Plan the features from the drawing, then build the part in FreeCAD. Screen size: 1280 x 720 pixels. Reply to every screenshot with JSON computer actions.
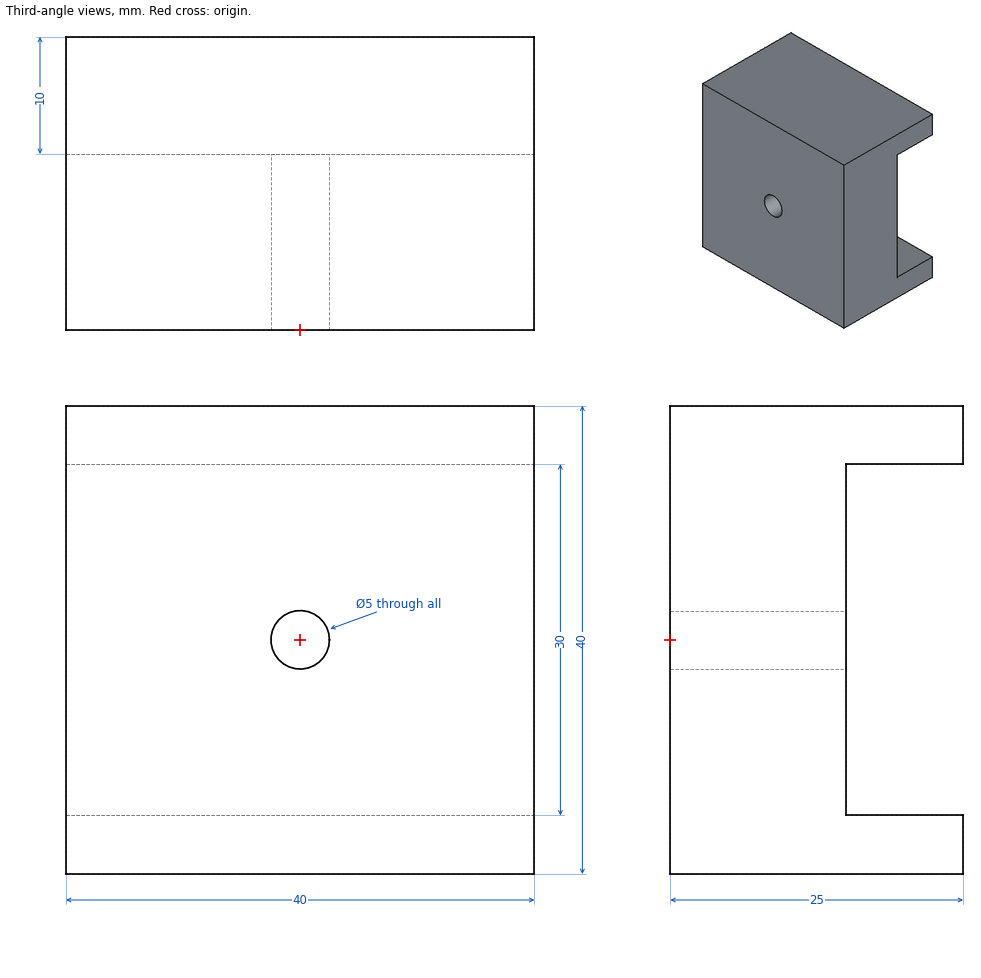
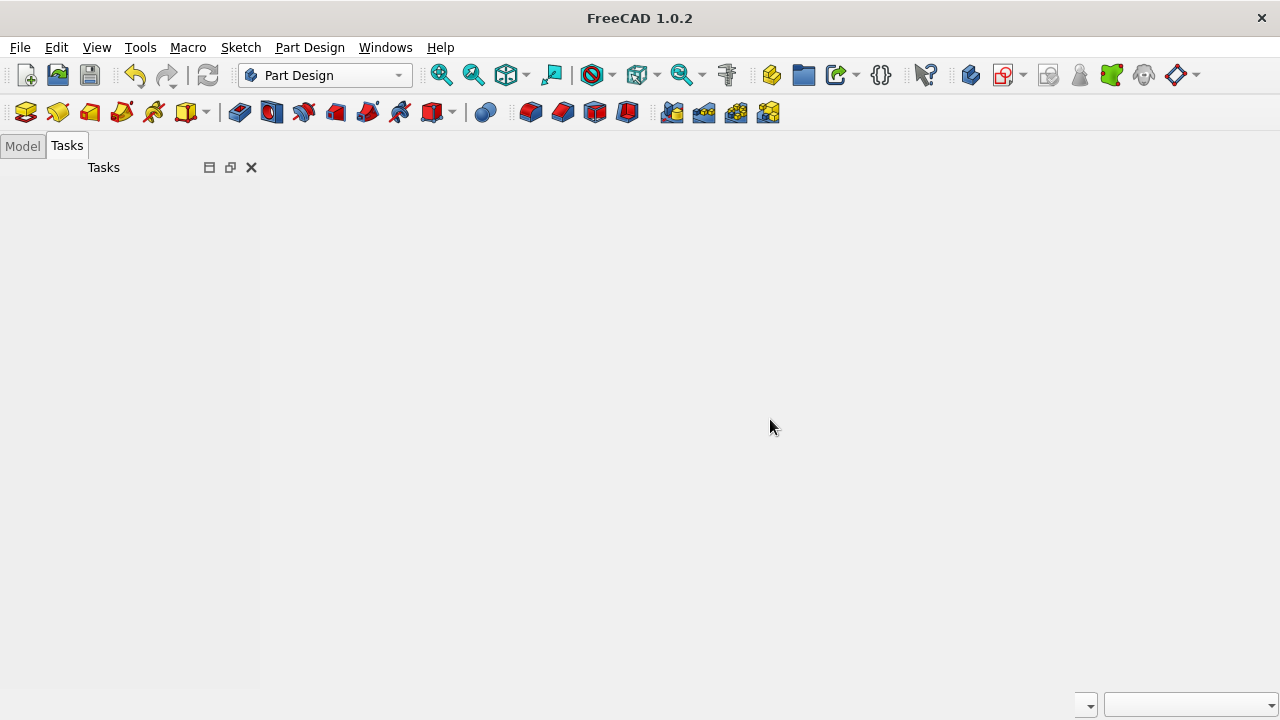
{"action": "left_click", "coordinate": [26, 76]}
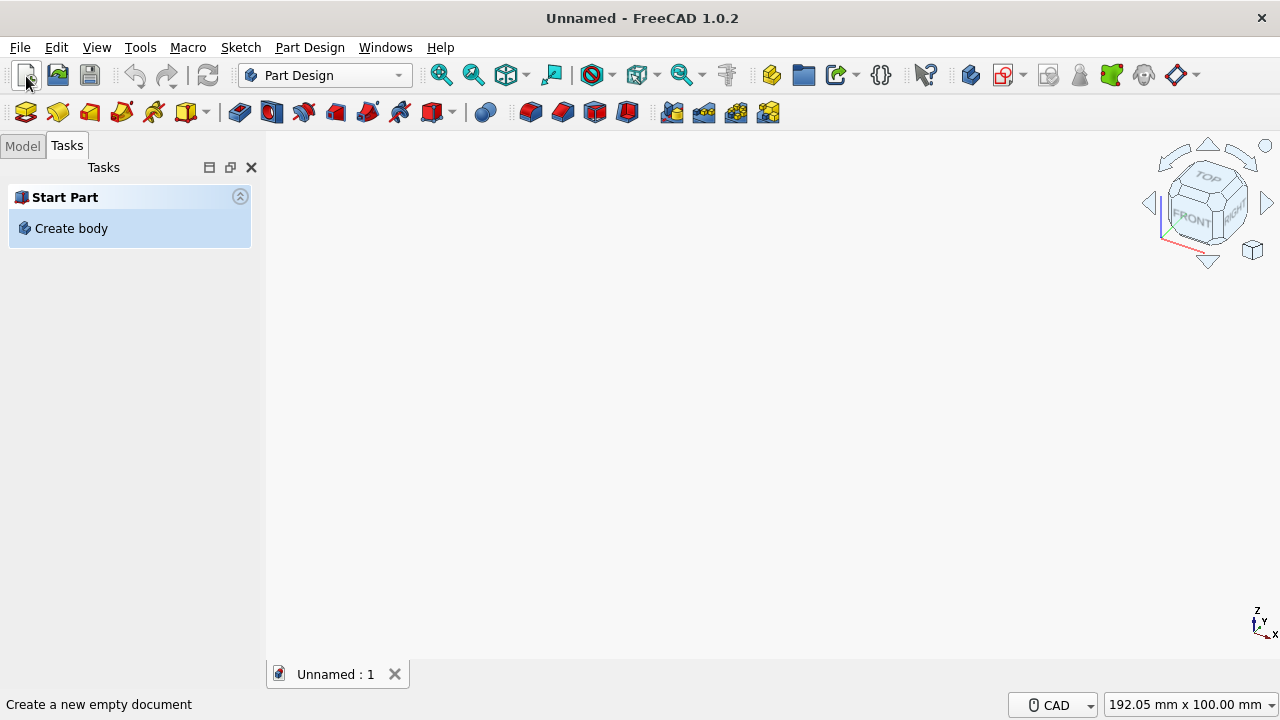
{"action": "left_click", "coordinate": [1004, 76]}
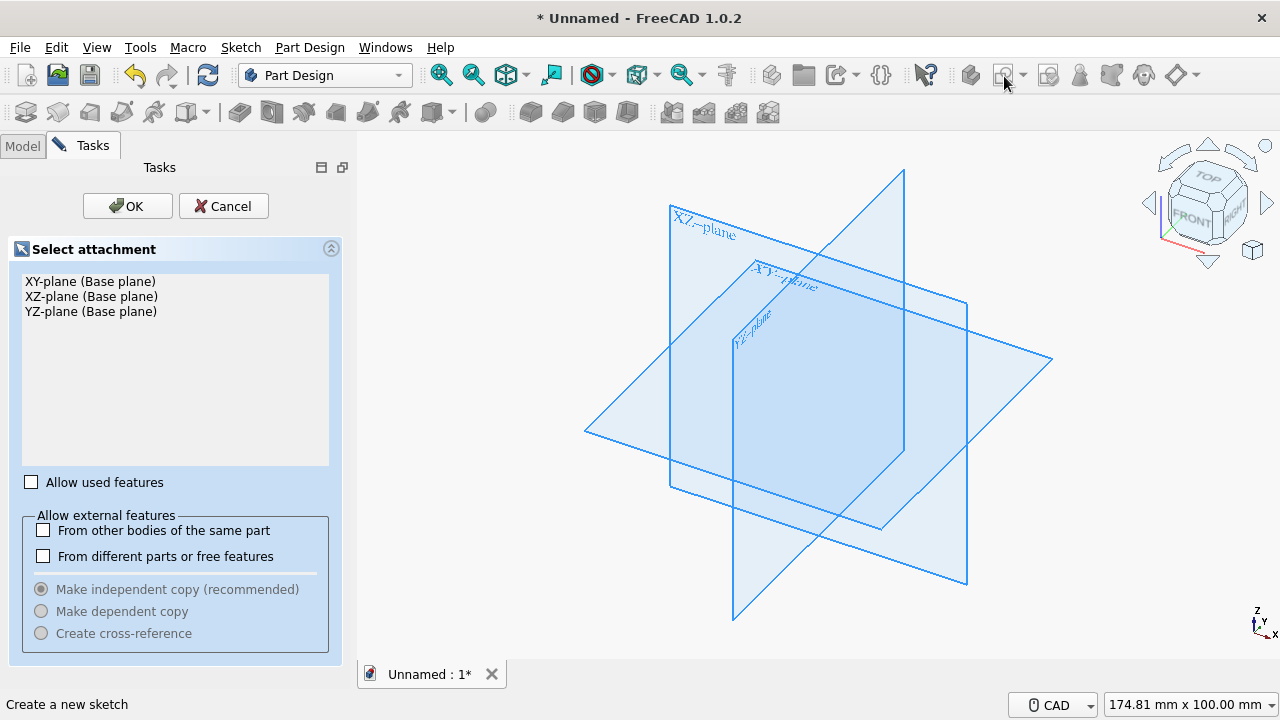
{"action": "left_click", "coordinate": [82, 296]}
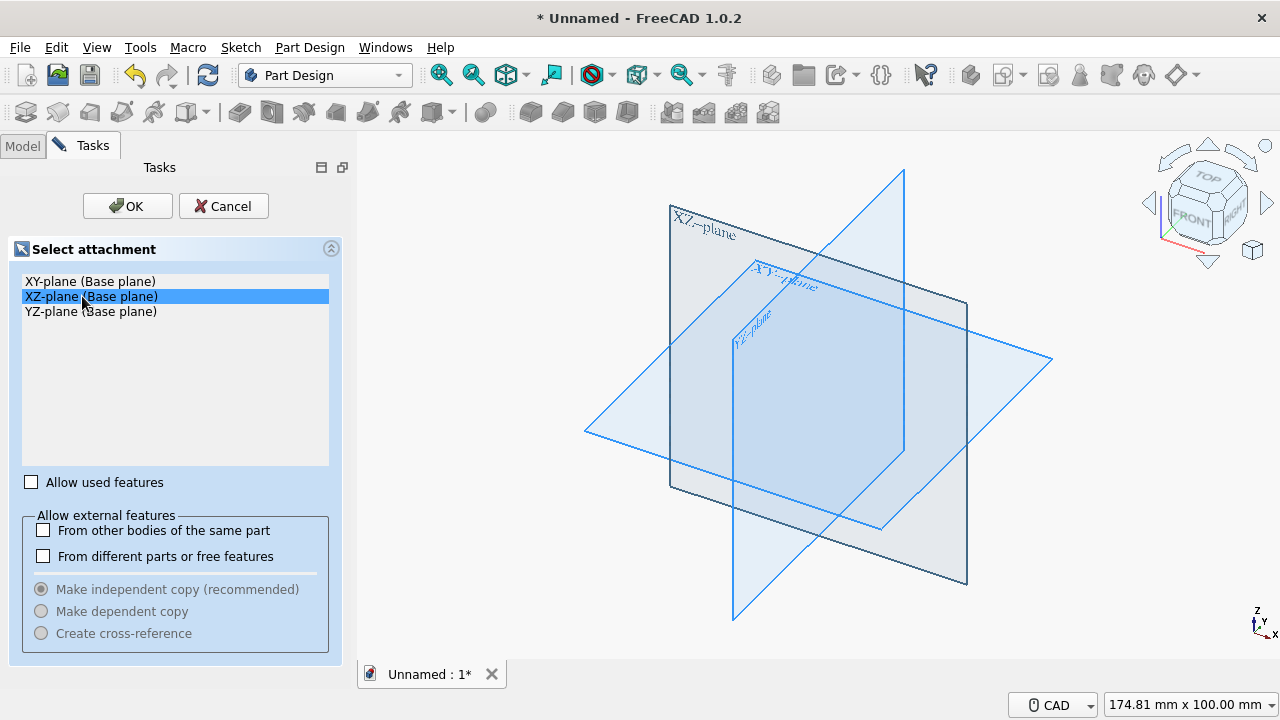
{"action": "left_click", "coordinate": [128, 206]}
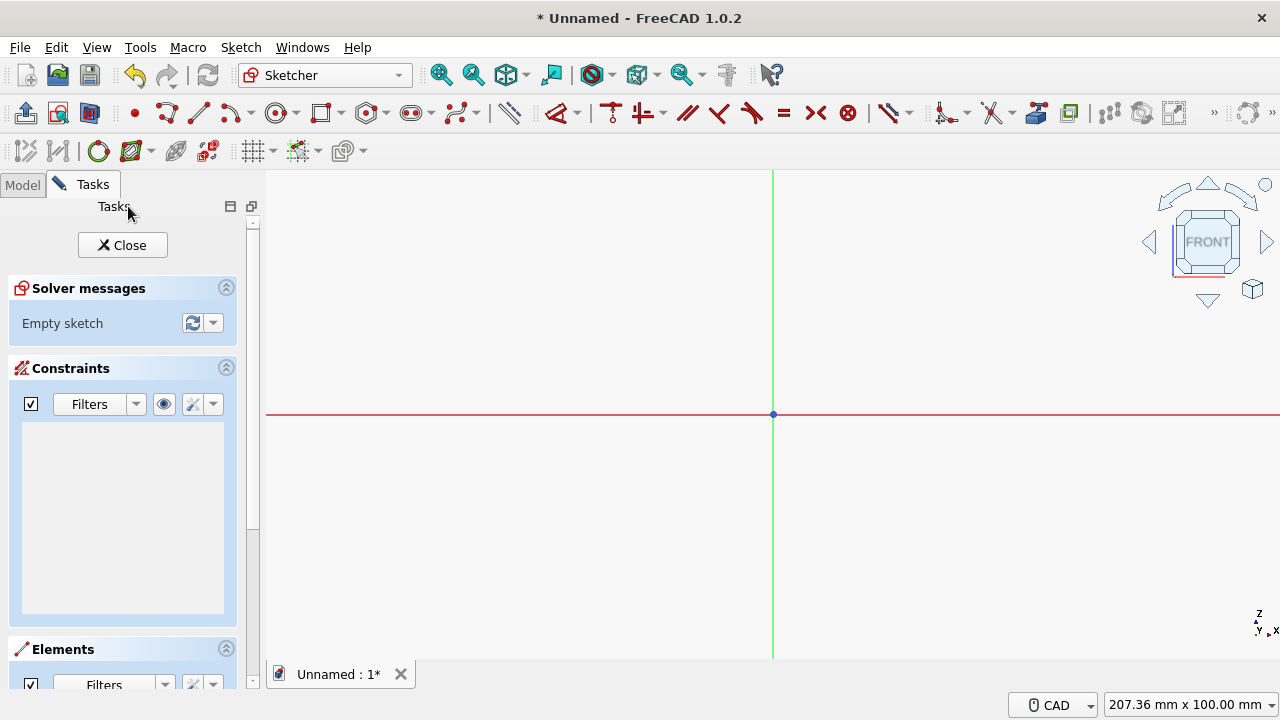
{"action": "scroll", "coordinate": [912, 414], "scroll_direction": "up", "scroll_amount": 2}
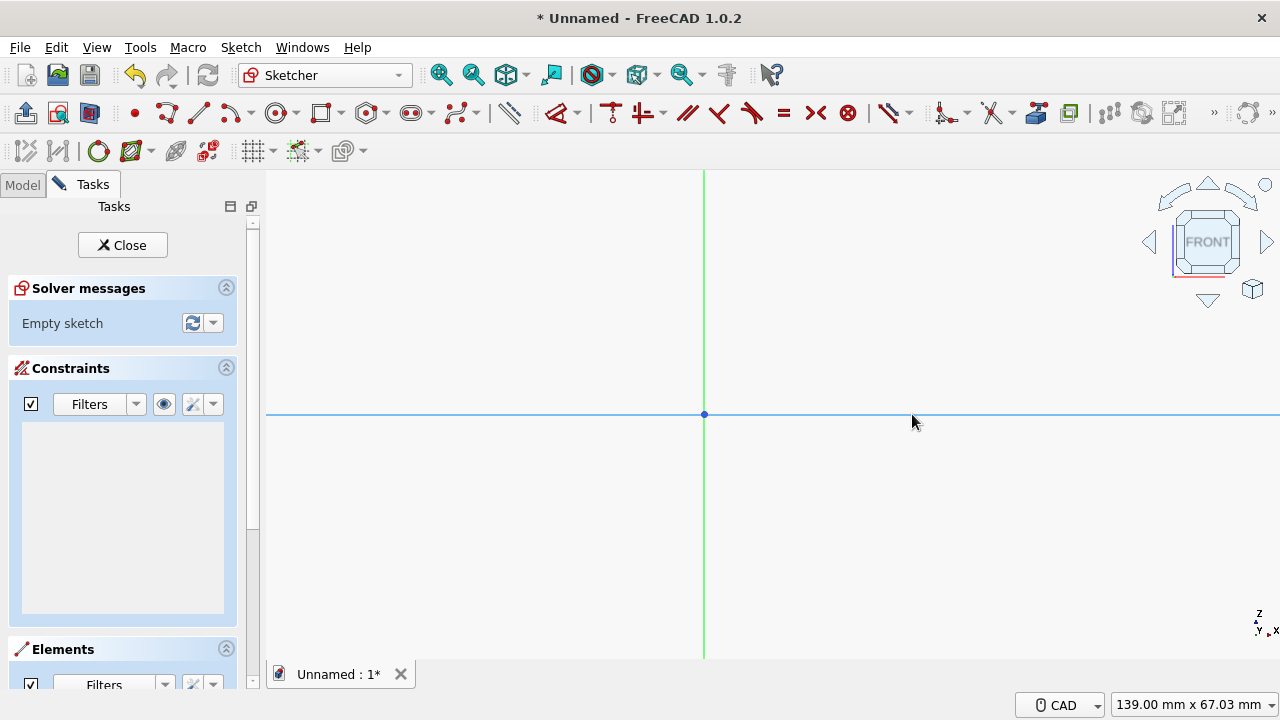
{"action": "key", "text": "g v"}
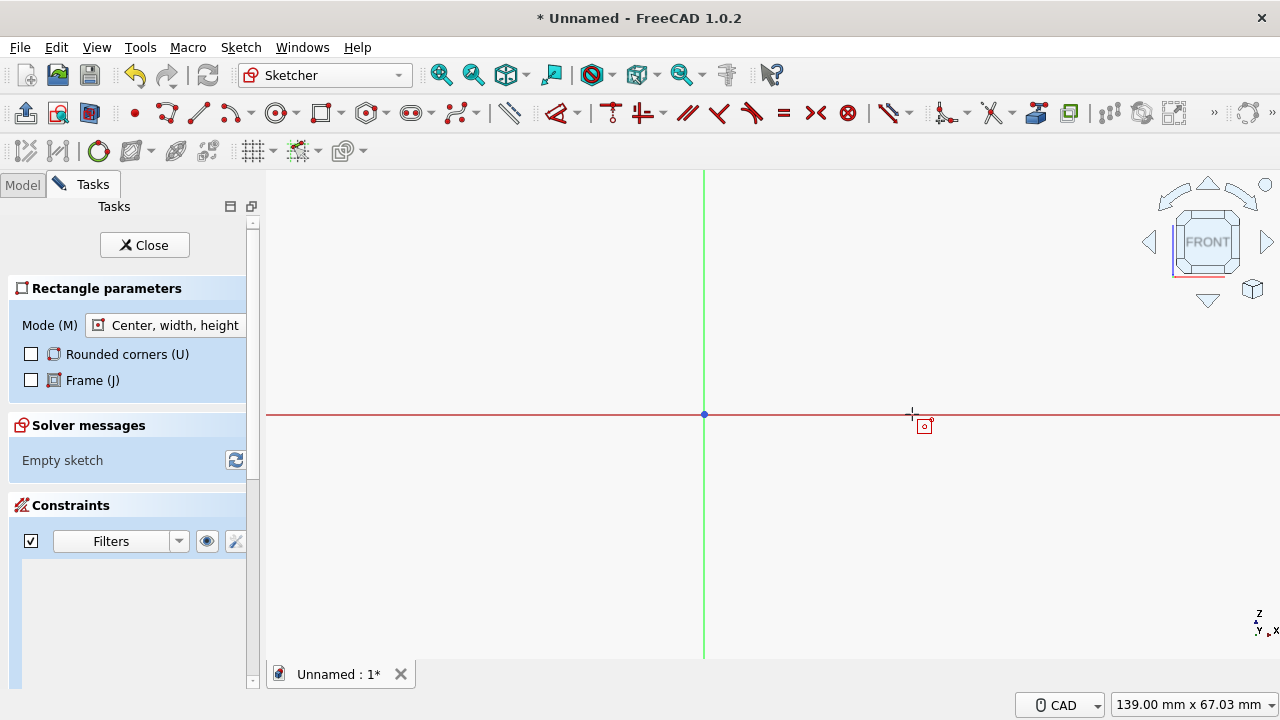
{"action": "left_click", "coordinate": [704, 414]}
{"action": "mouse_move", "coordinate": [850, 269]}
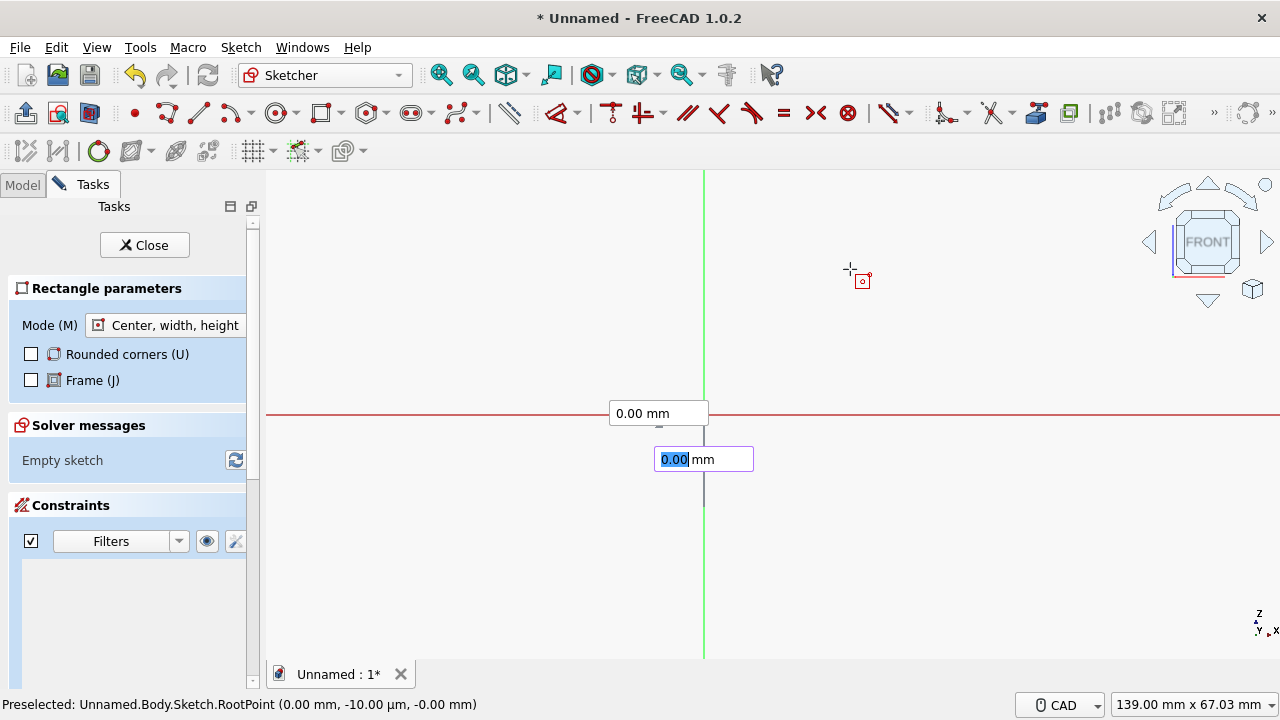
{"action": "type", "text": "40"}
{"action": "key", "text": "Tab"}
{"action": "type", "text": "40"}
{"action": "key", "text": "Return"}
{"action": "key", "text": "Escape"}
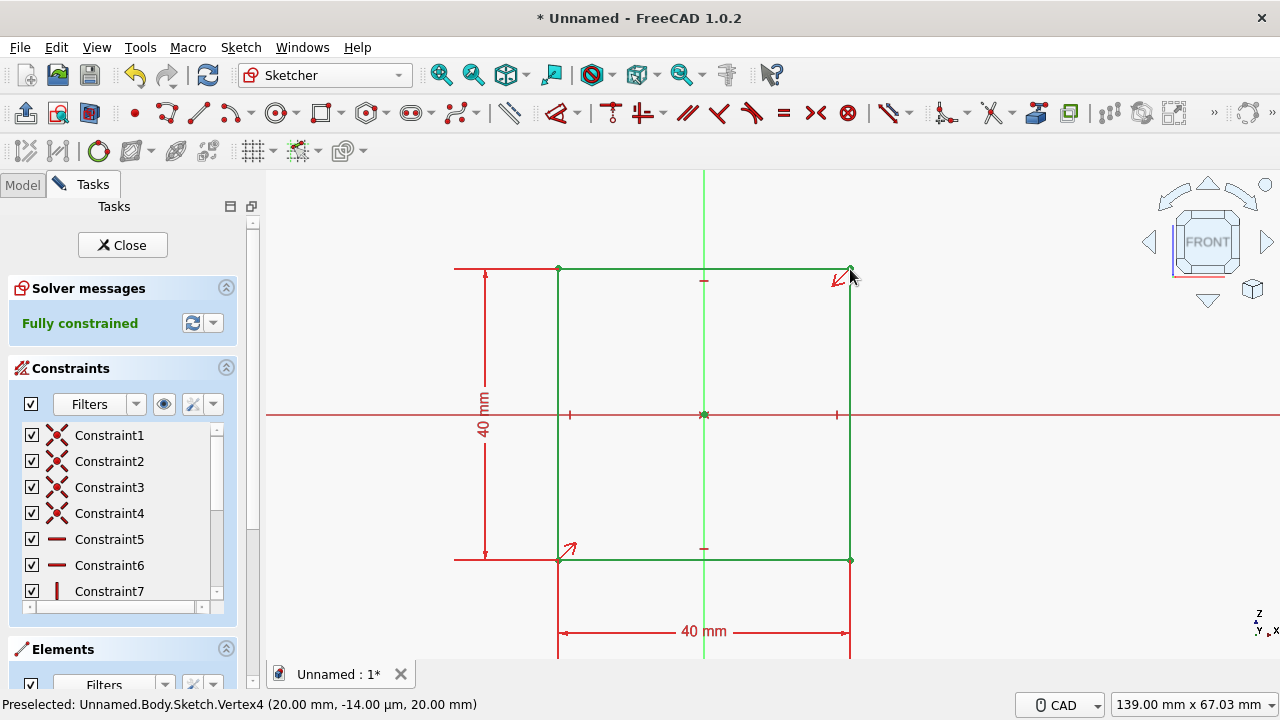
{"action": "left_click", "coordinate": [123, 245]}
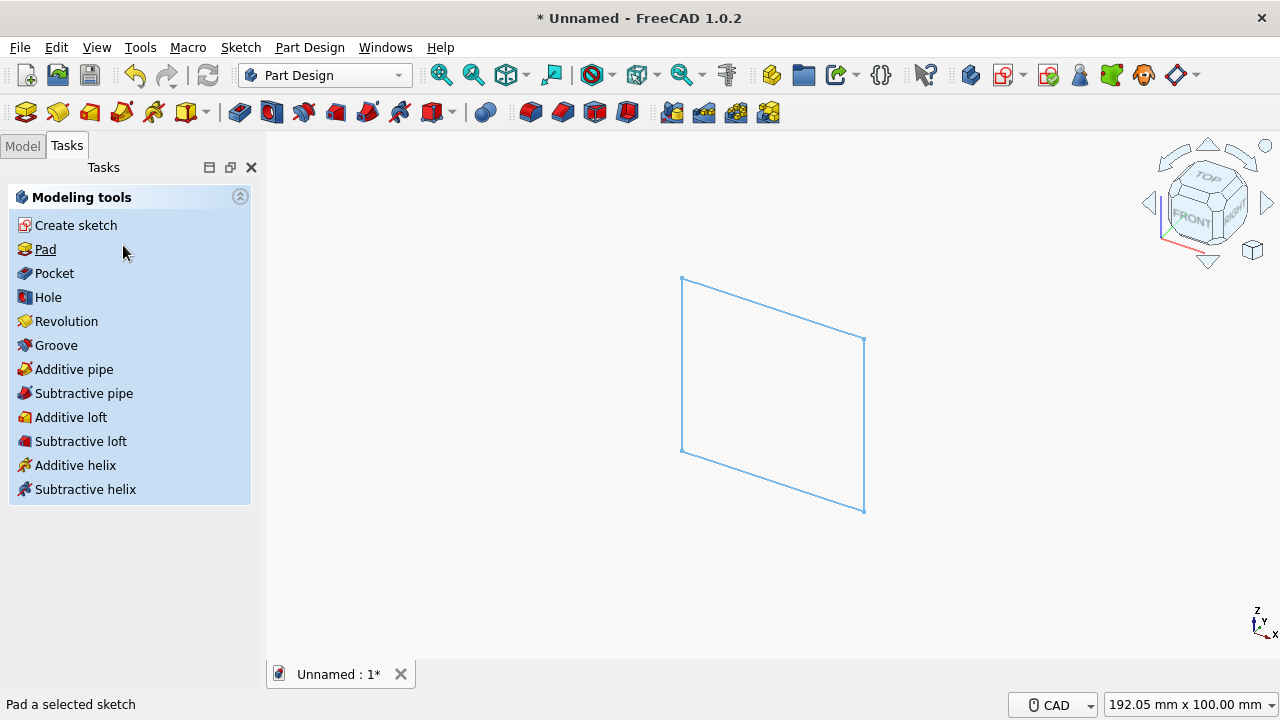
{"action": "left_click", "coordinate": [26, 112]}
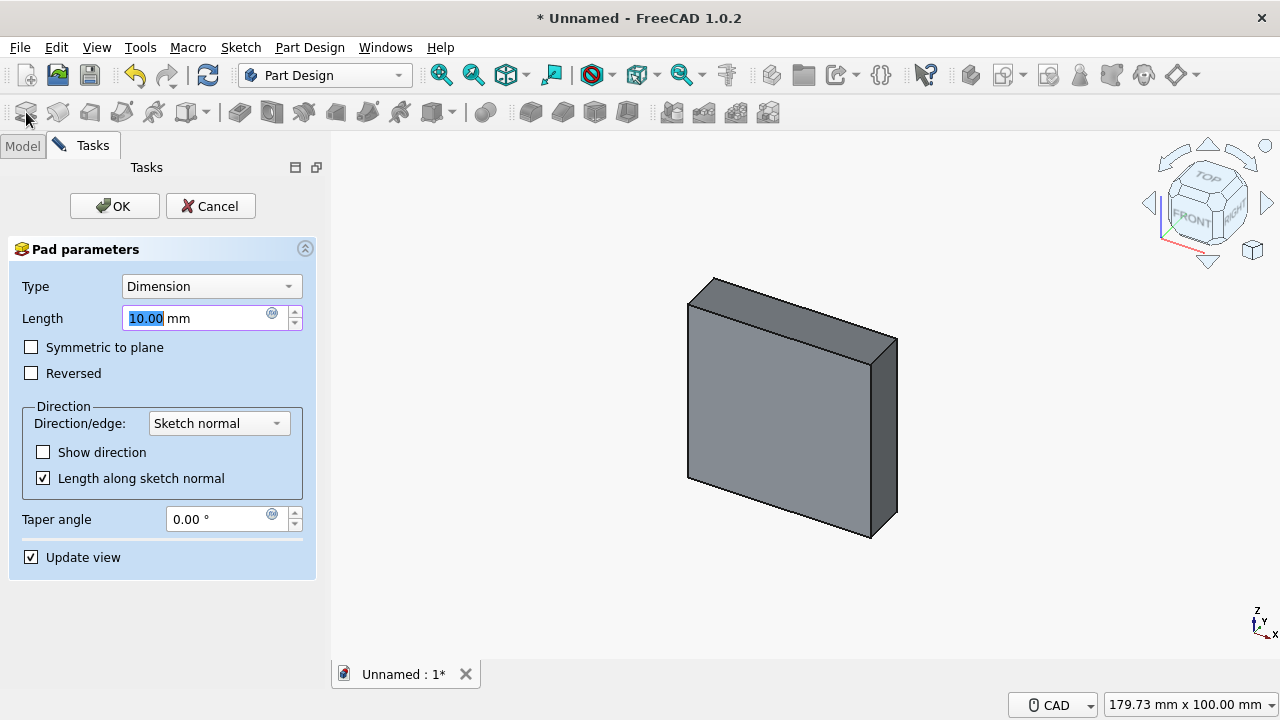
{"action": "type", "text": "25"}
{"action": "key", "text": "Tab"}